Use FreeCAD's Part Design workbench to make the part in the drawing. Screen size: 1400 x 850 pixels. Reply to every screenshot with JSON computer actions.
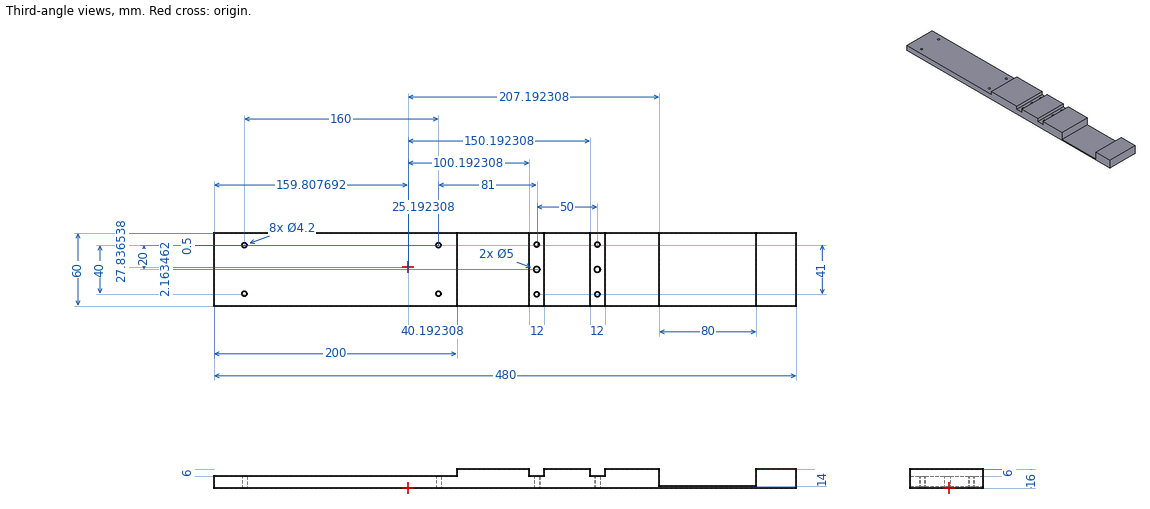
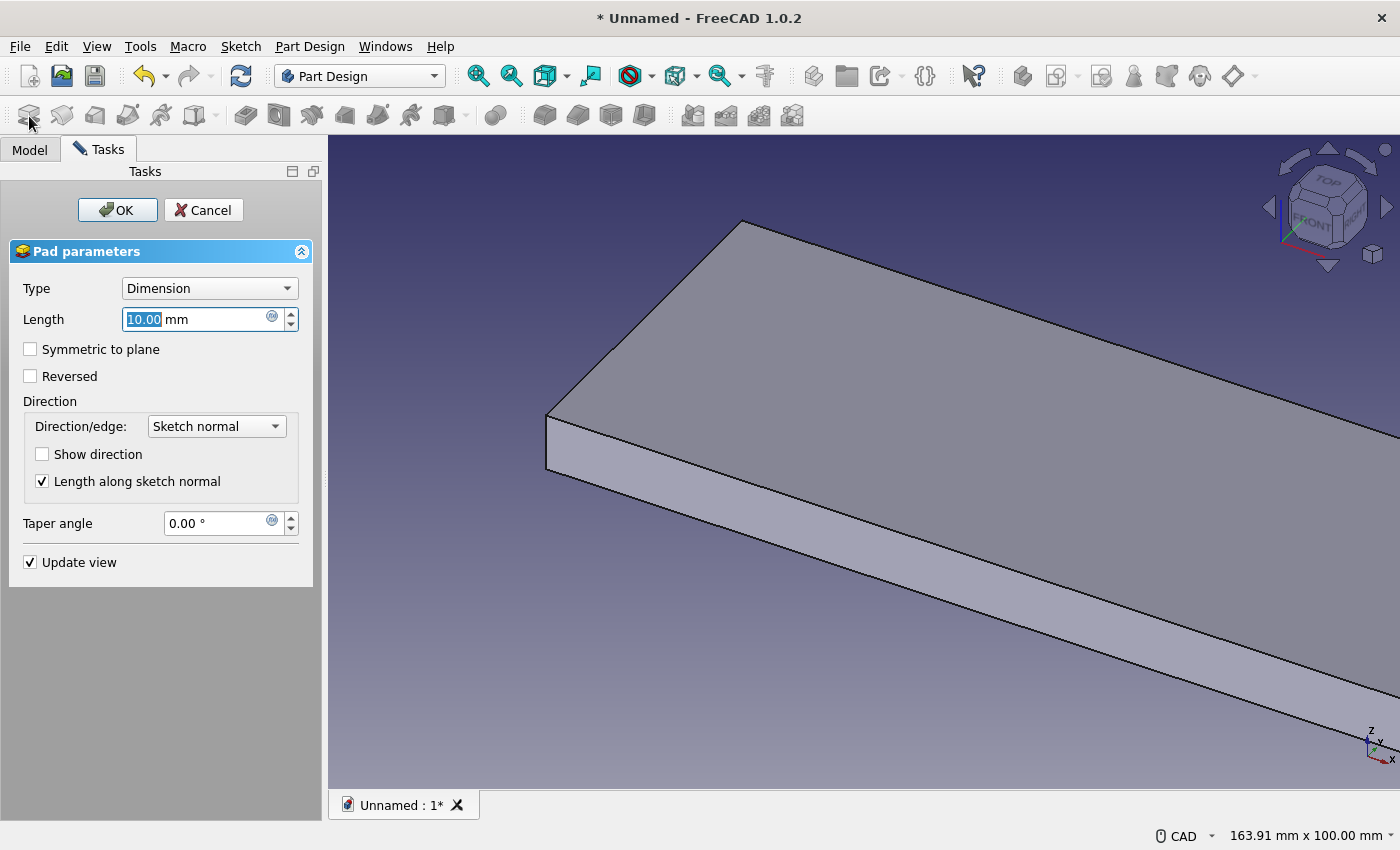
{"action": "type", "text": "16"}
{"action": "key", "text": "Tab"}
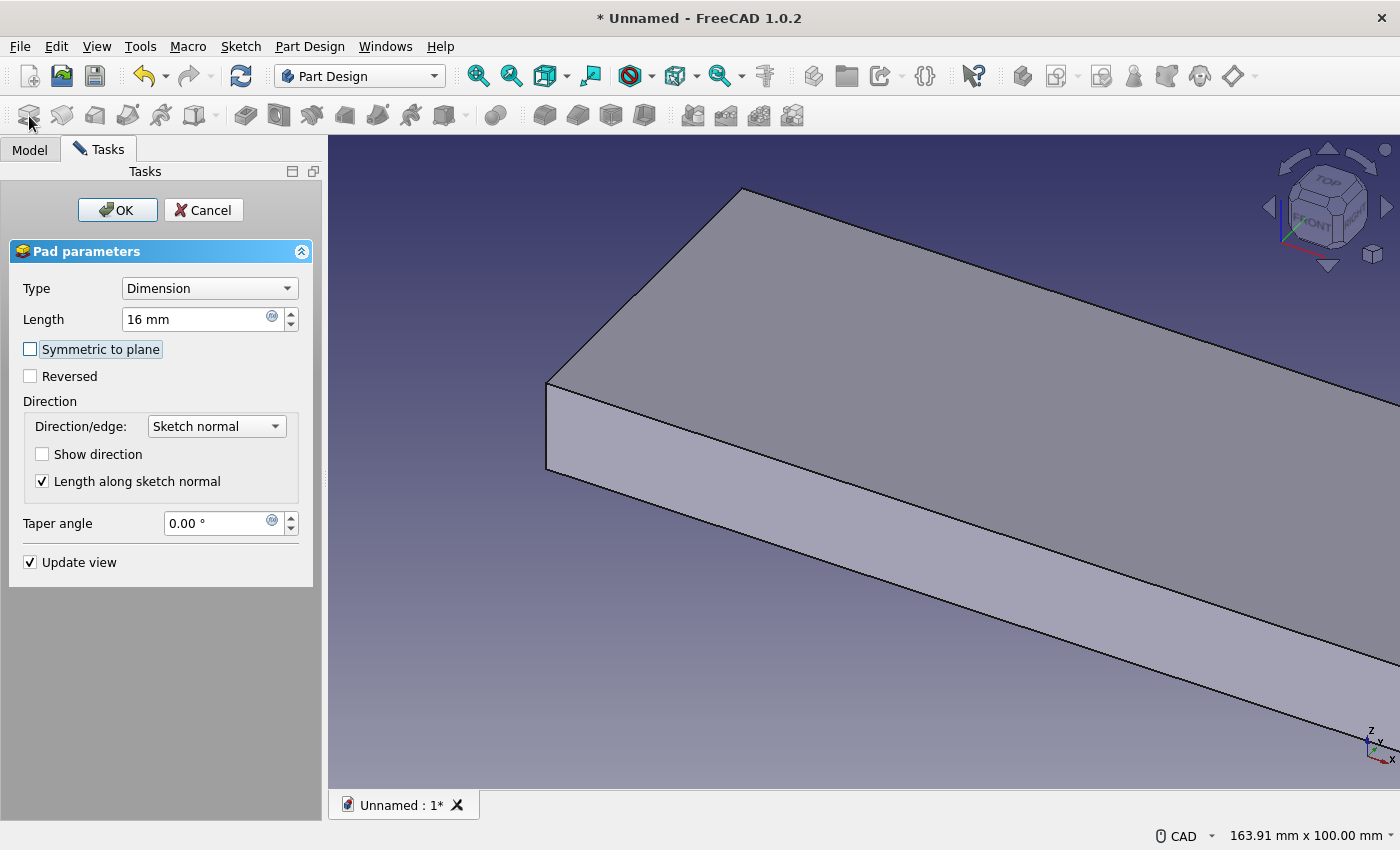
{"action": "left_click", "coordinate": [118, 210]}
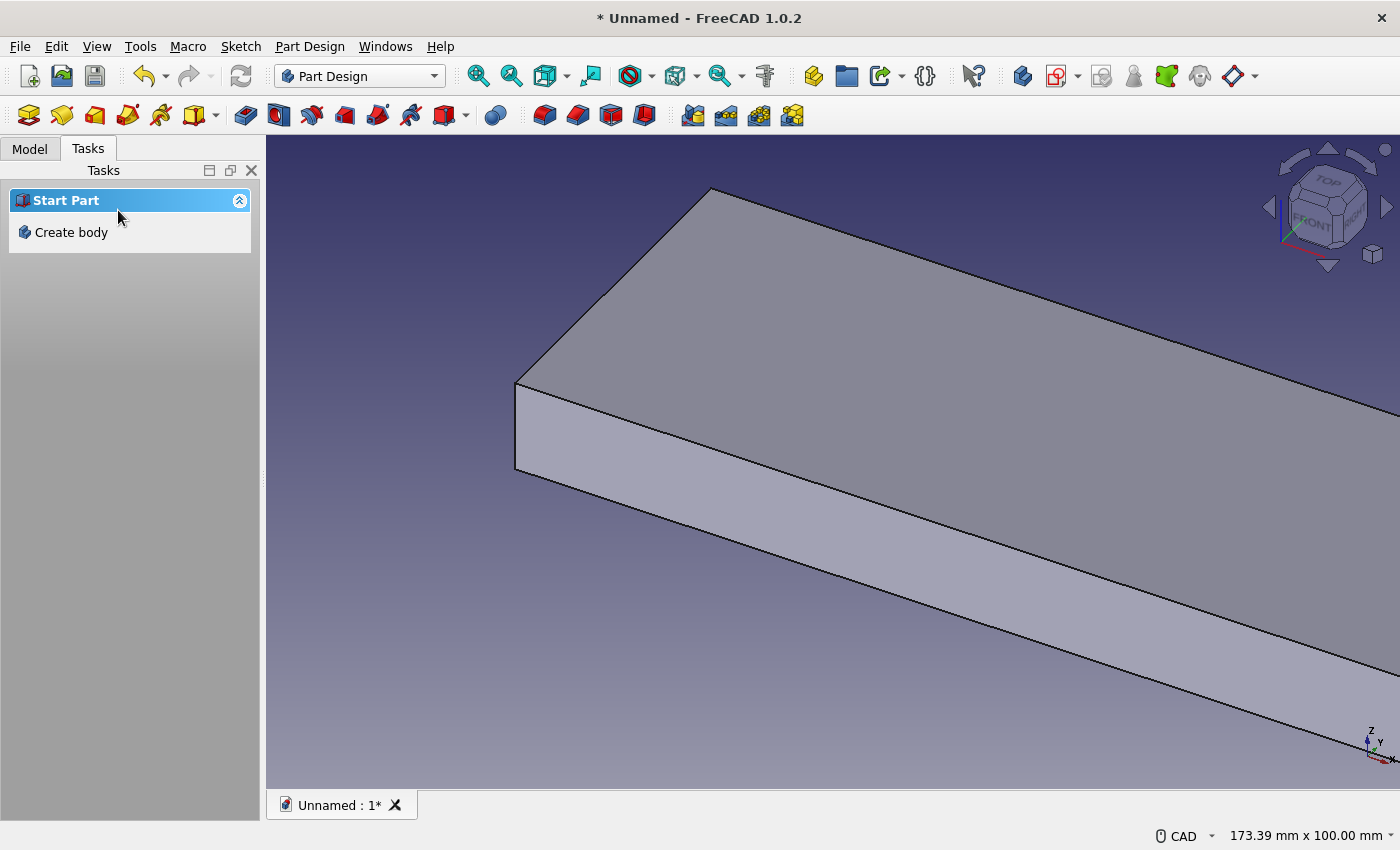
{"action": "left_click", "coordinate": [479, 76]}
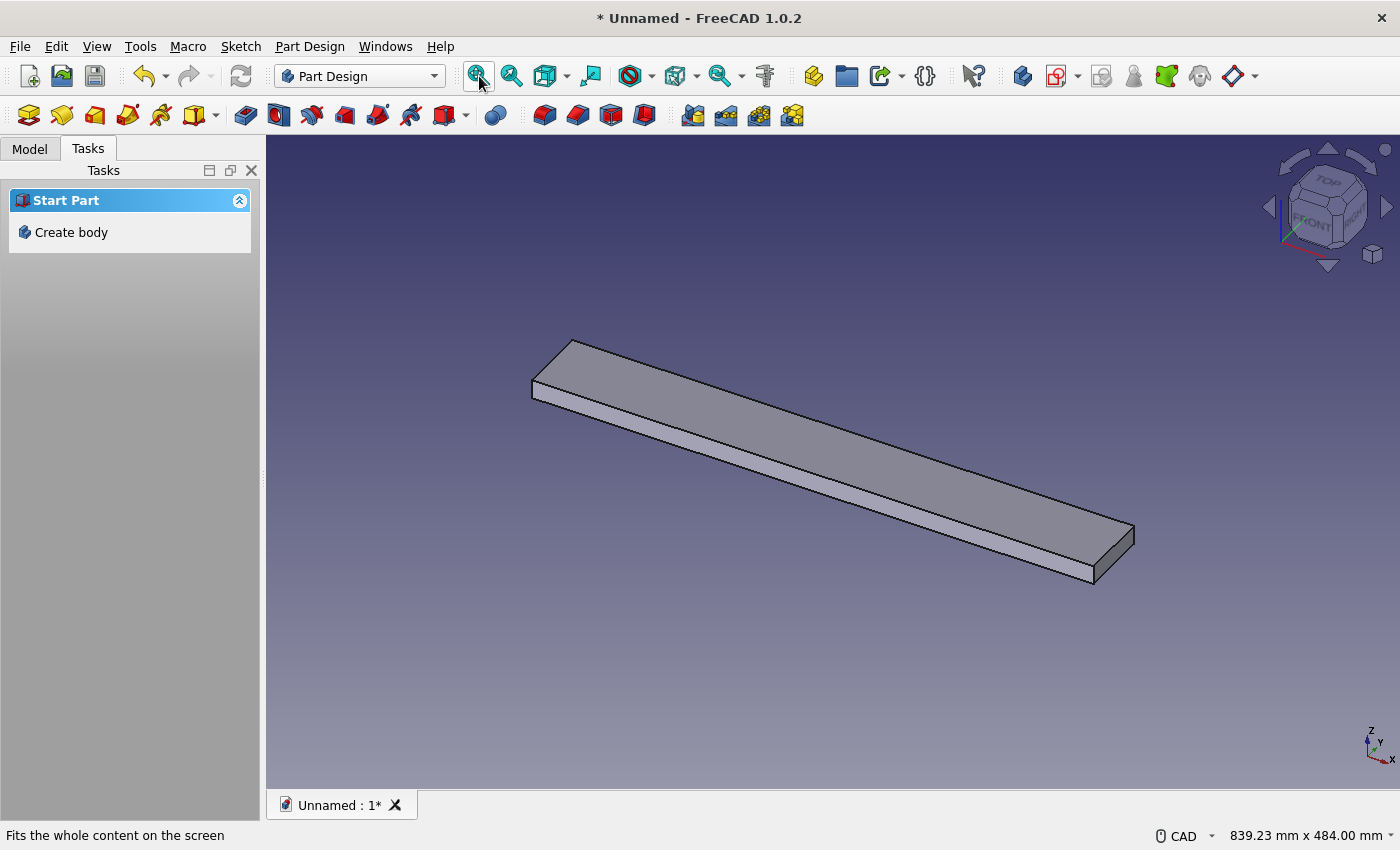
{"action": "left_click", "coordinate": [1074, 532]}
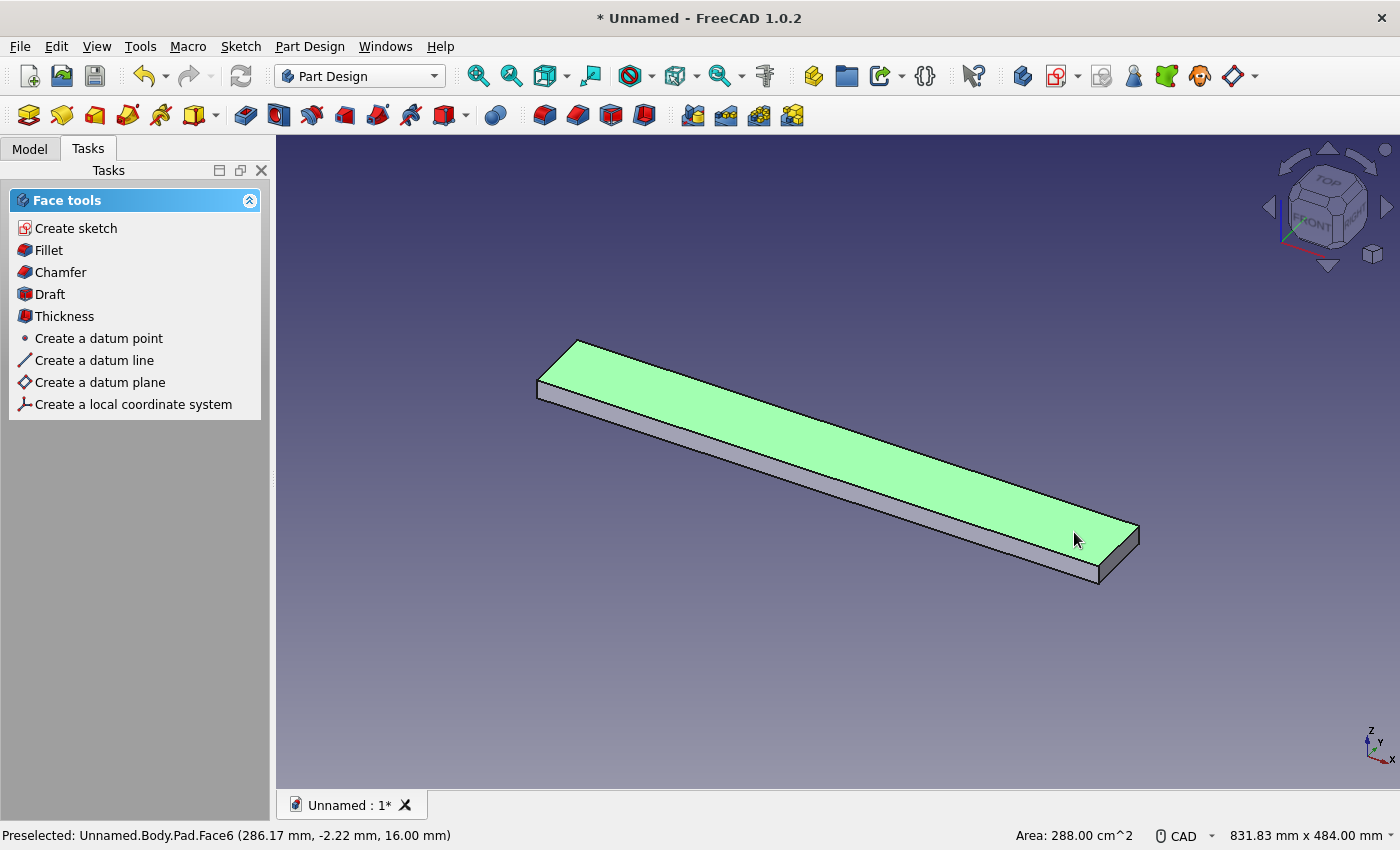
{"action": "left_click", "coordinate": [1056, 76]}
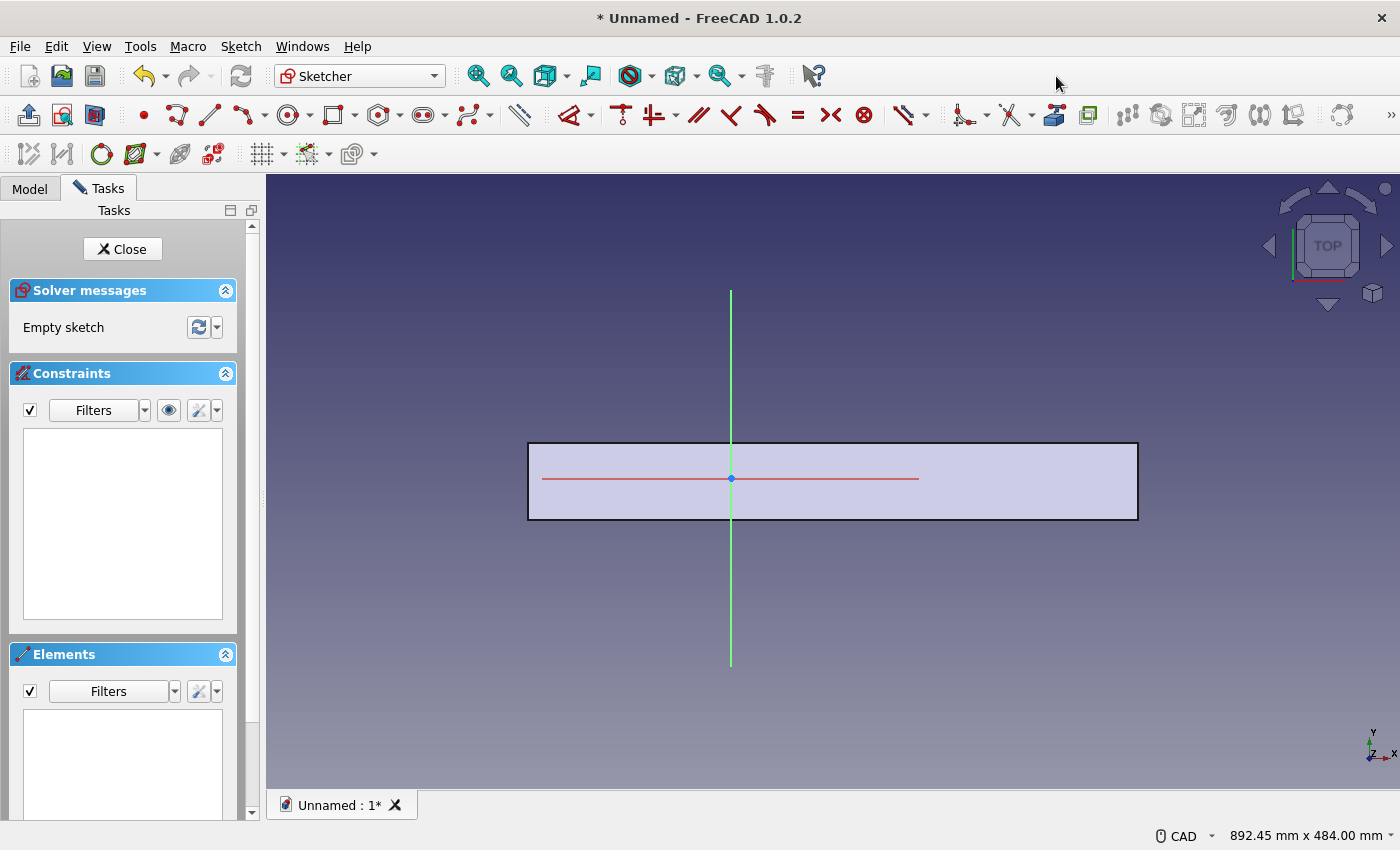
{"action": "scroll", "coordinate": [591, 481], "scroll_direction": "up", "scroll_amount": 5}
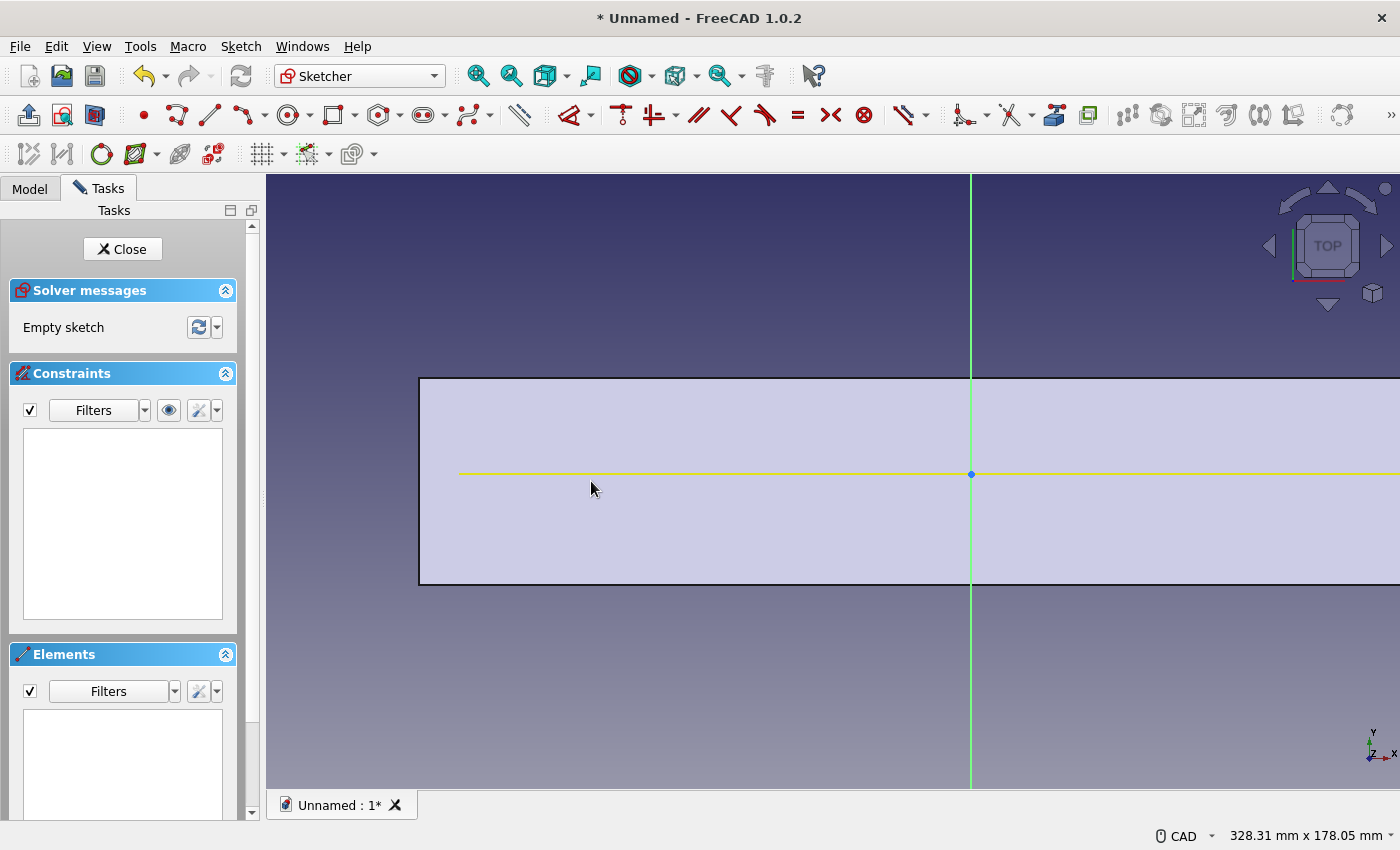
{"action": "left_click", "coordinate": [332, 116]}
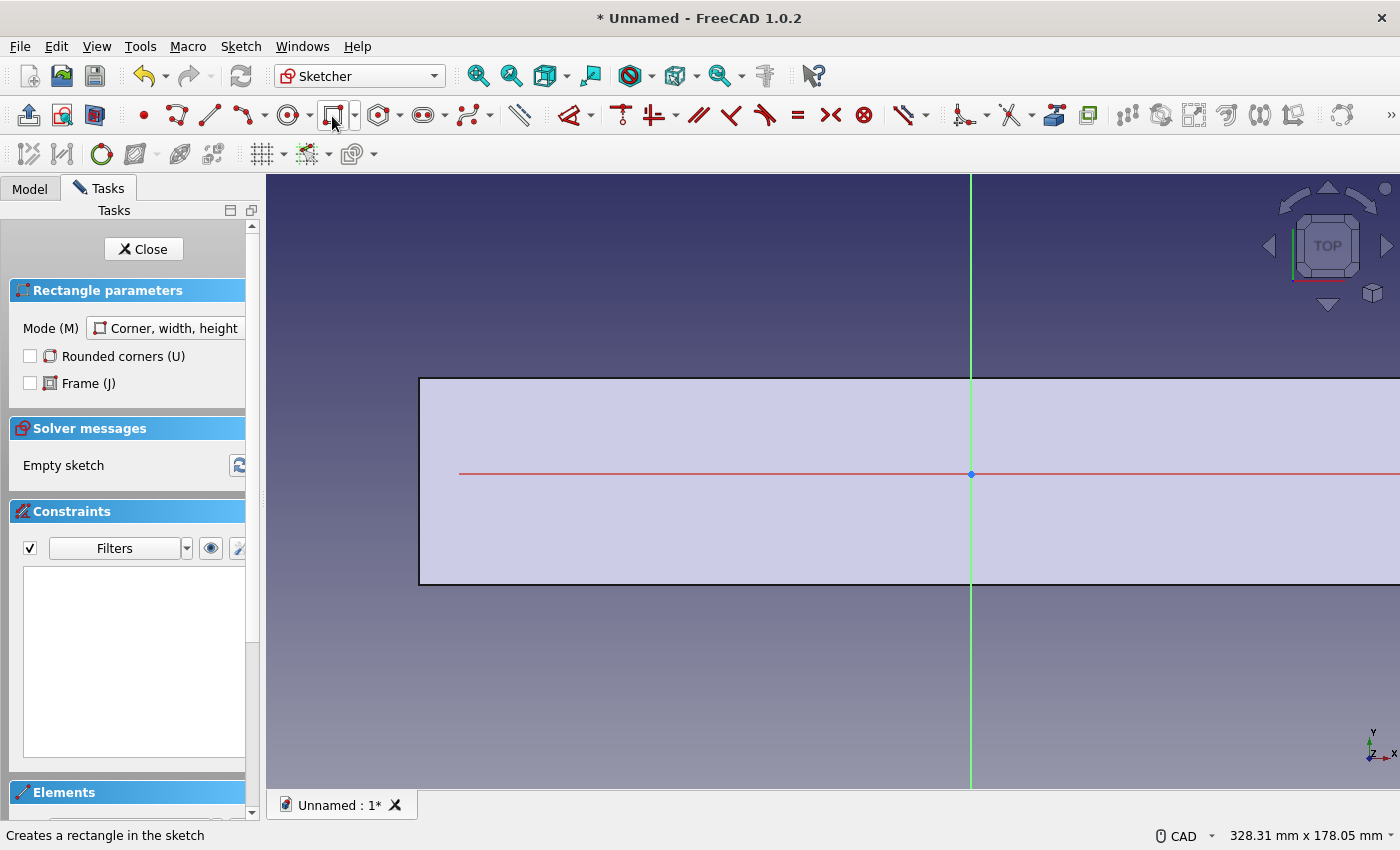
{"action": "left_click", "coordinate": [419, 378]}
{"action": "left_click", "coordinate": [1110, 585]}
{"action": "key", "text": "Escape"}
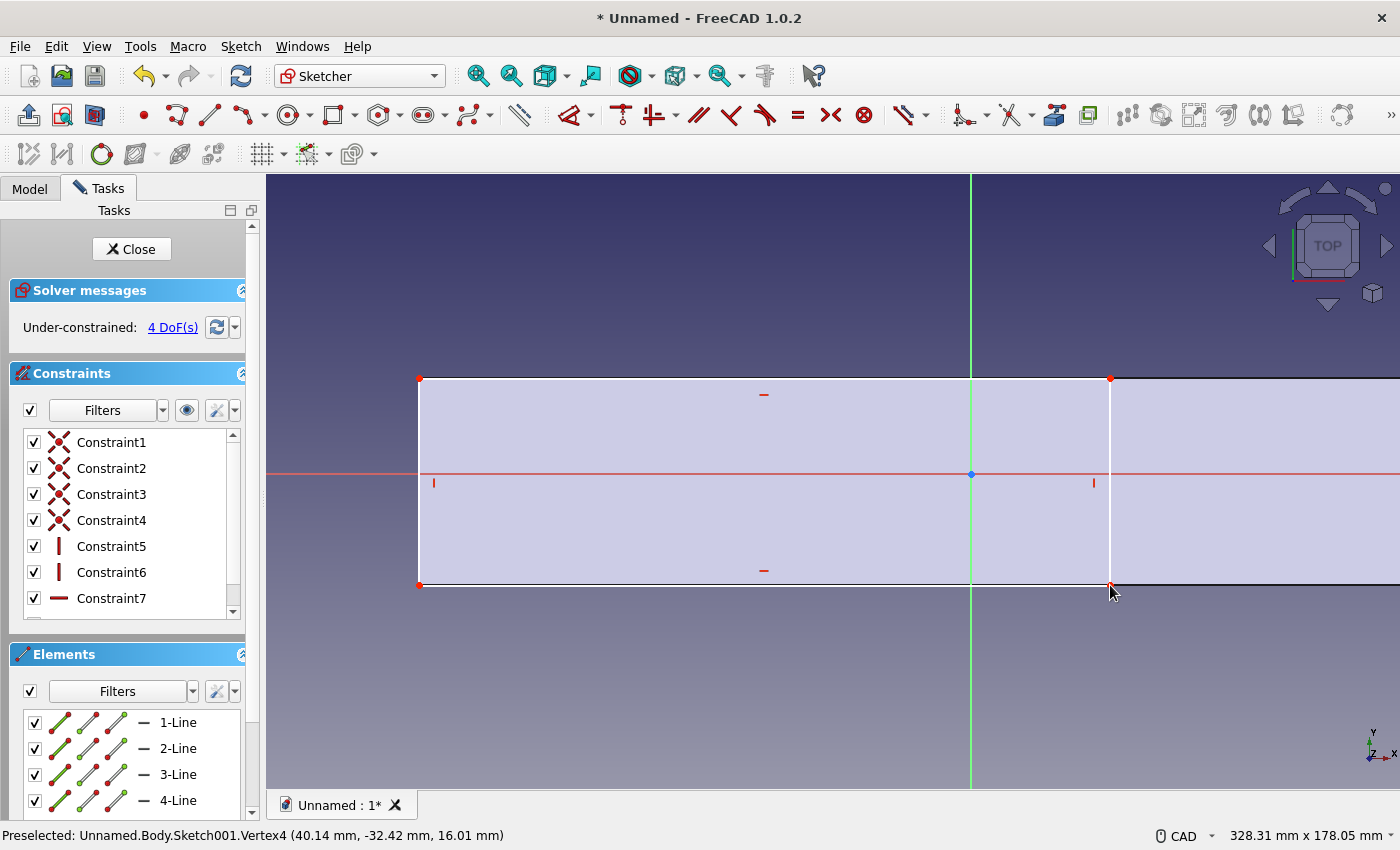
{"action": "left_click", "coordinate": [568, 116]}